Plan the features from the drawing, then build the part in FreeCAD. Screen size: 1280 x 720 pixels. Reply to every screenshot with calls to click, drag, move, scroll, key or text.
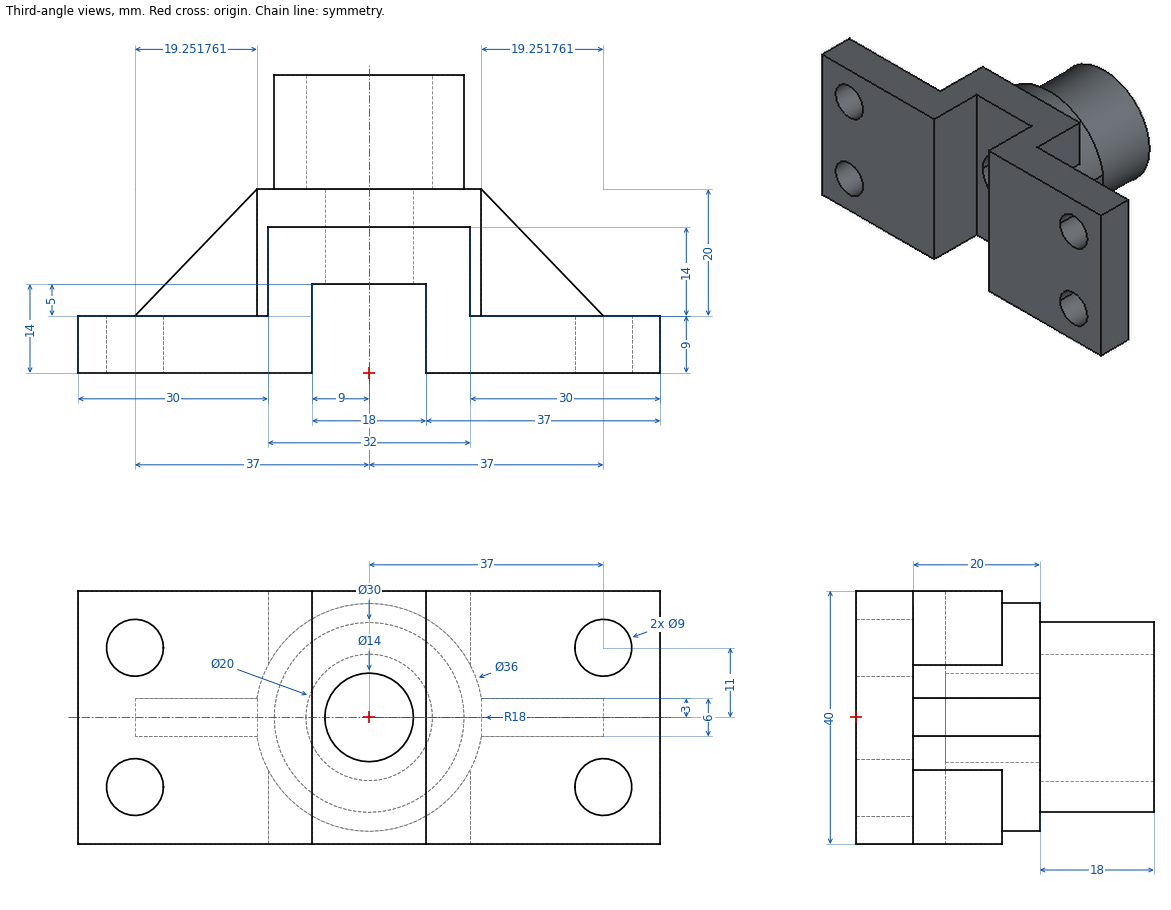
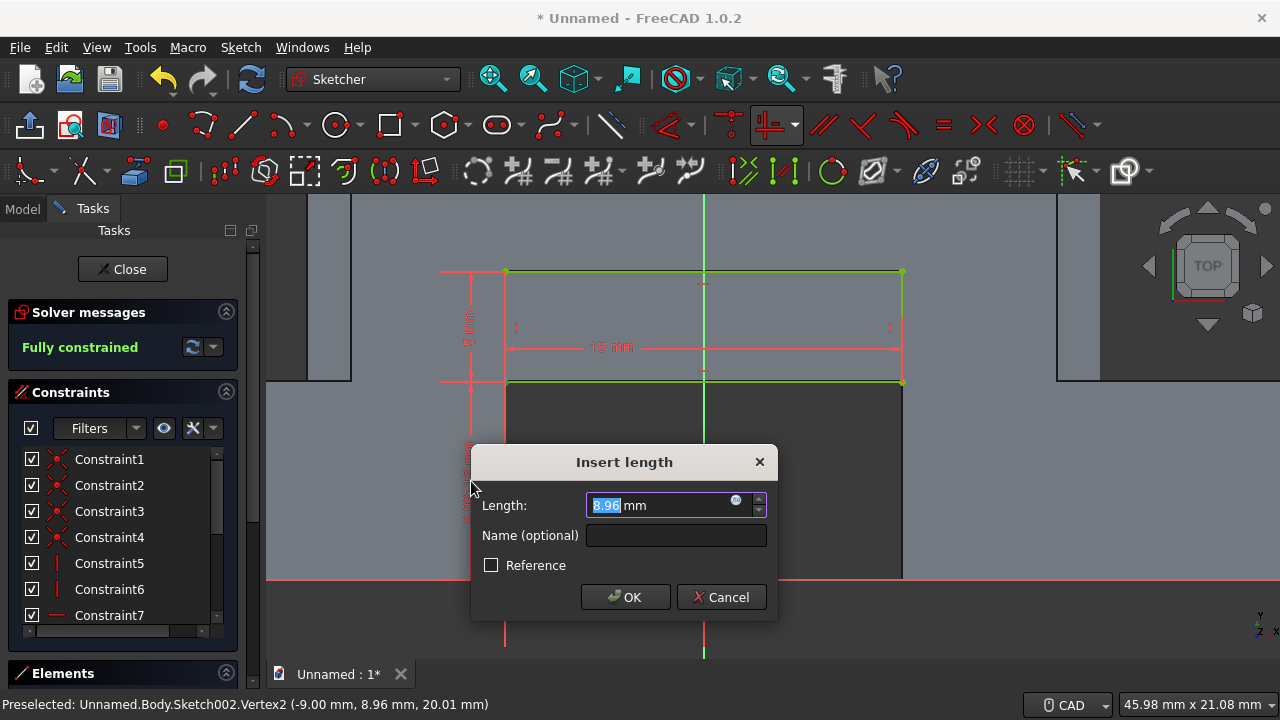
text(9)
key(Return)
key(Escape)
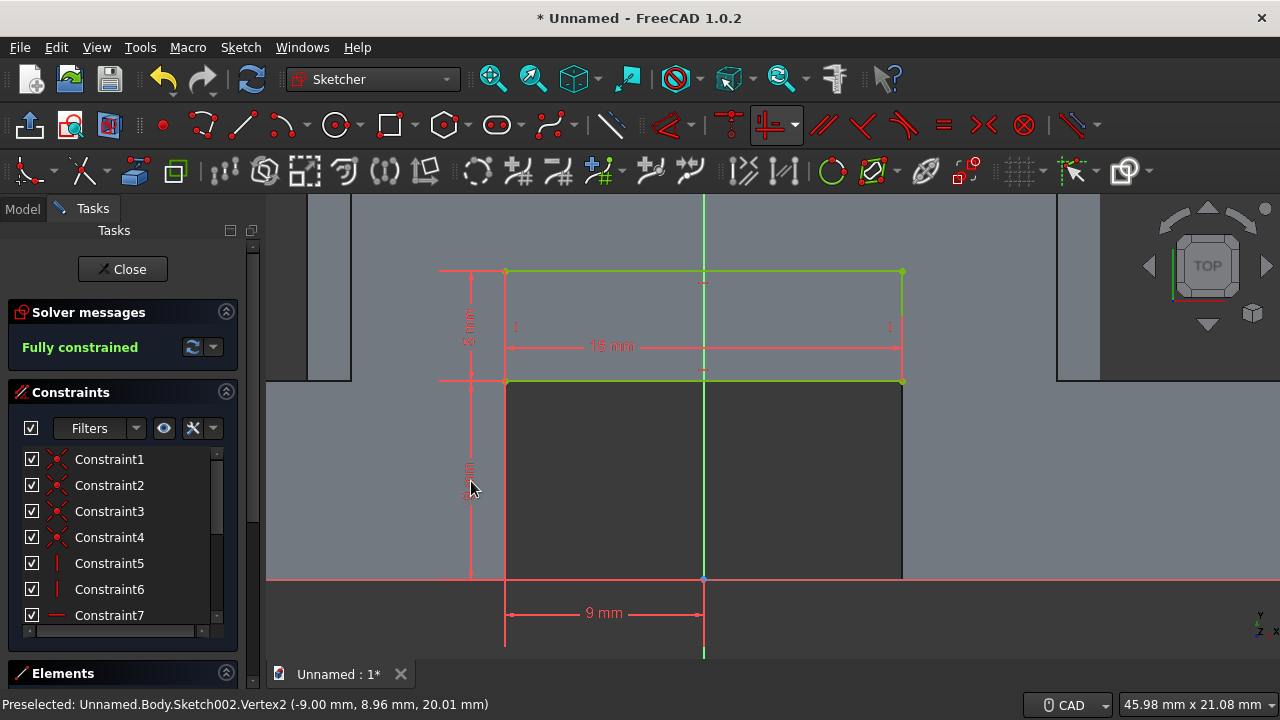
click(123, 269)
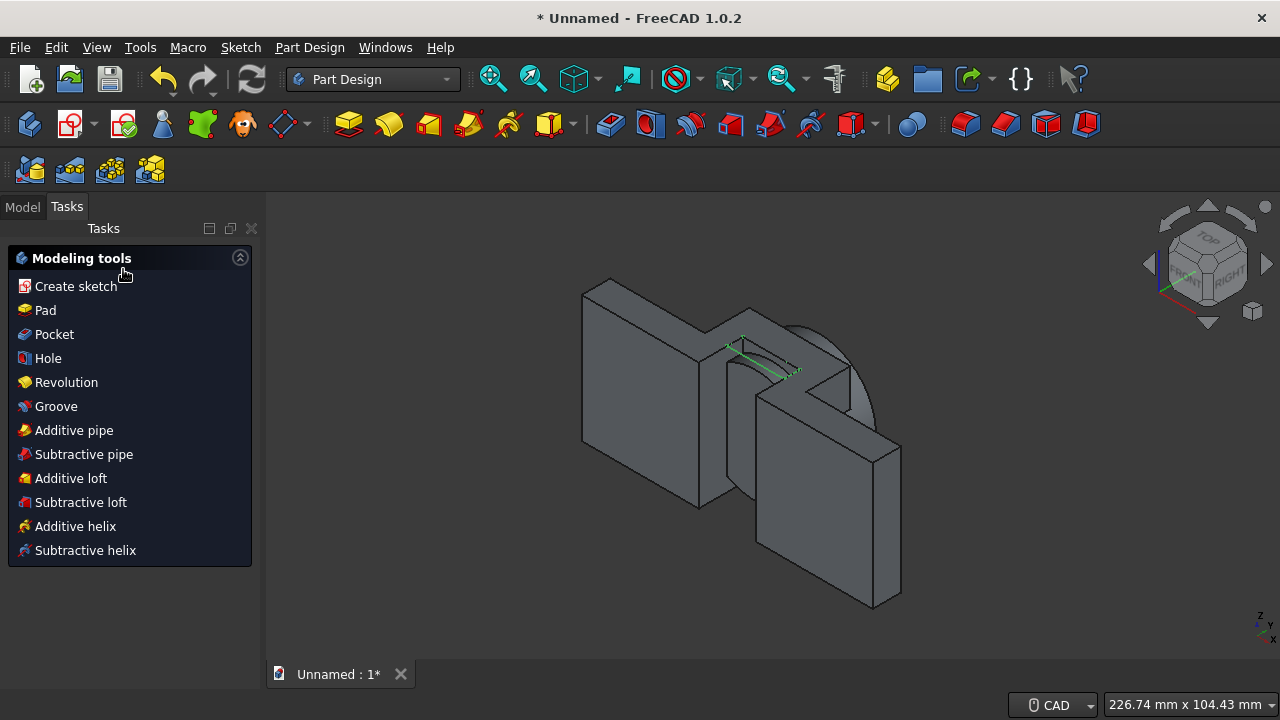
click(612, 124)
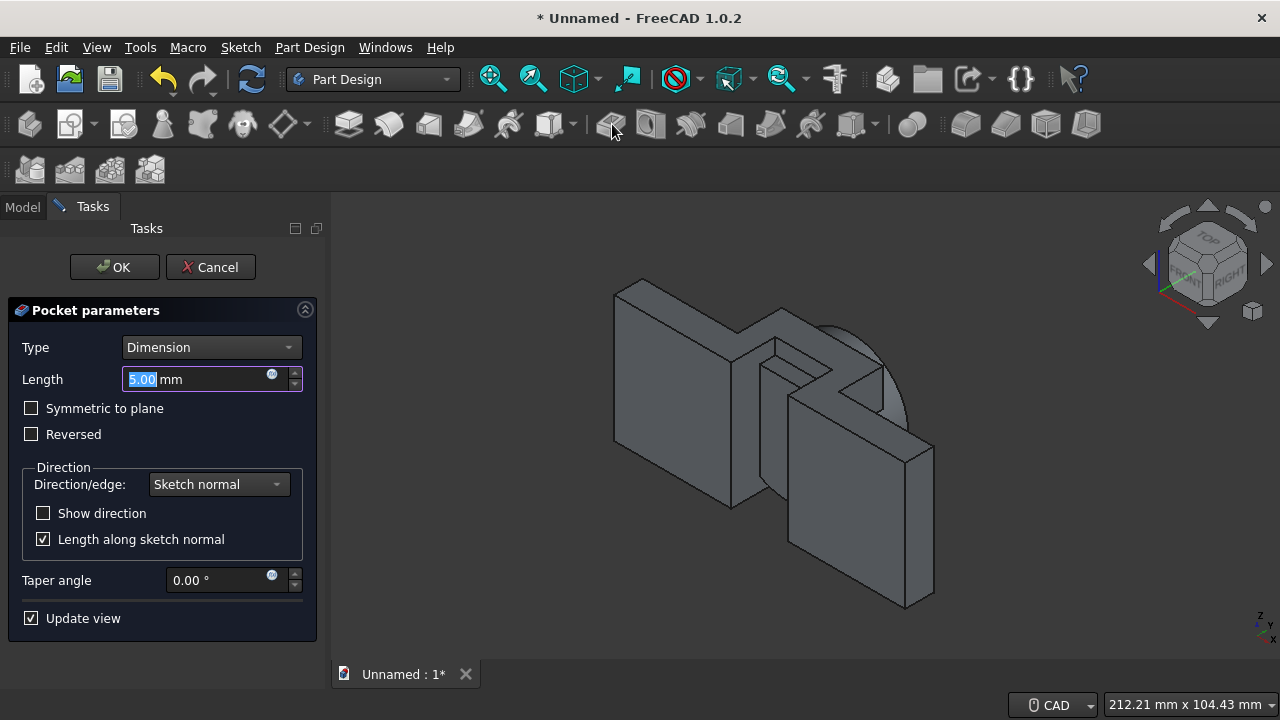
click(212, 348)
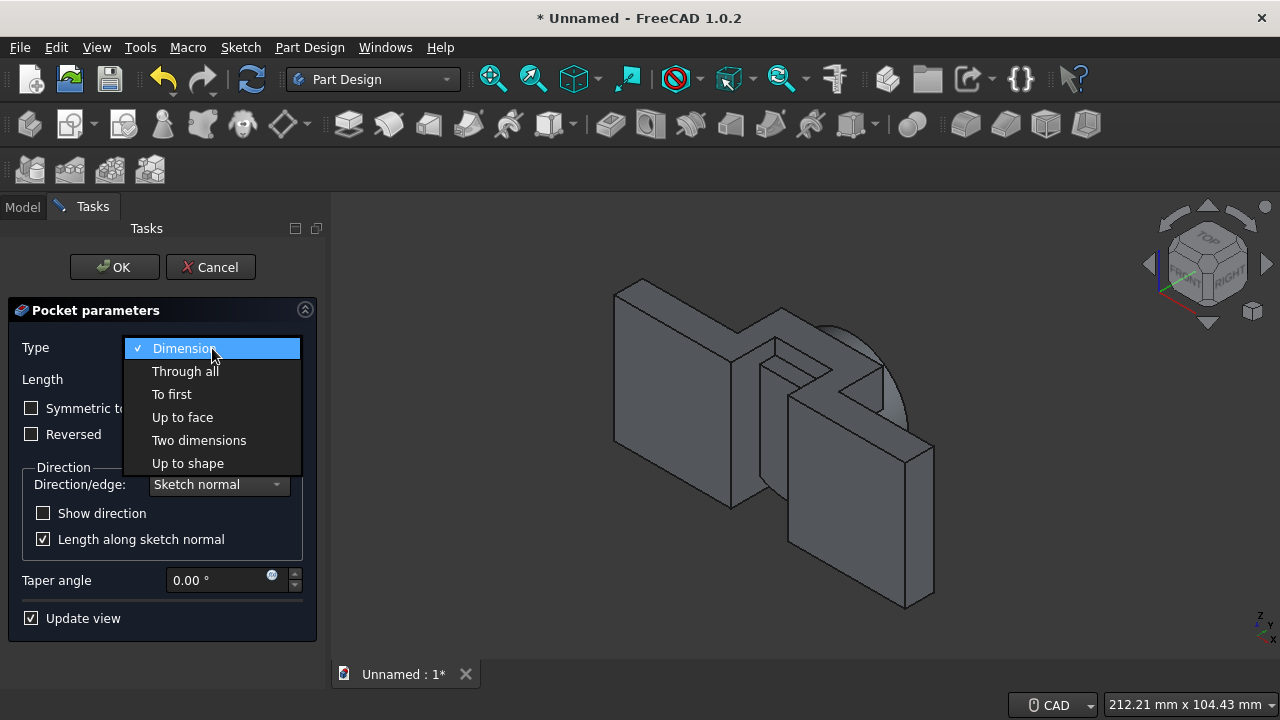
click(212, 372)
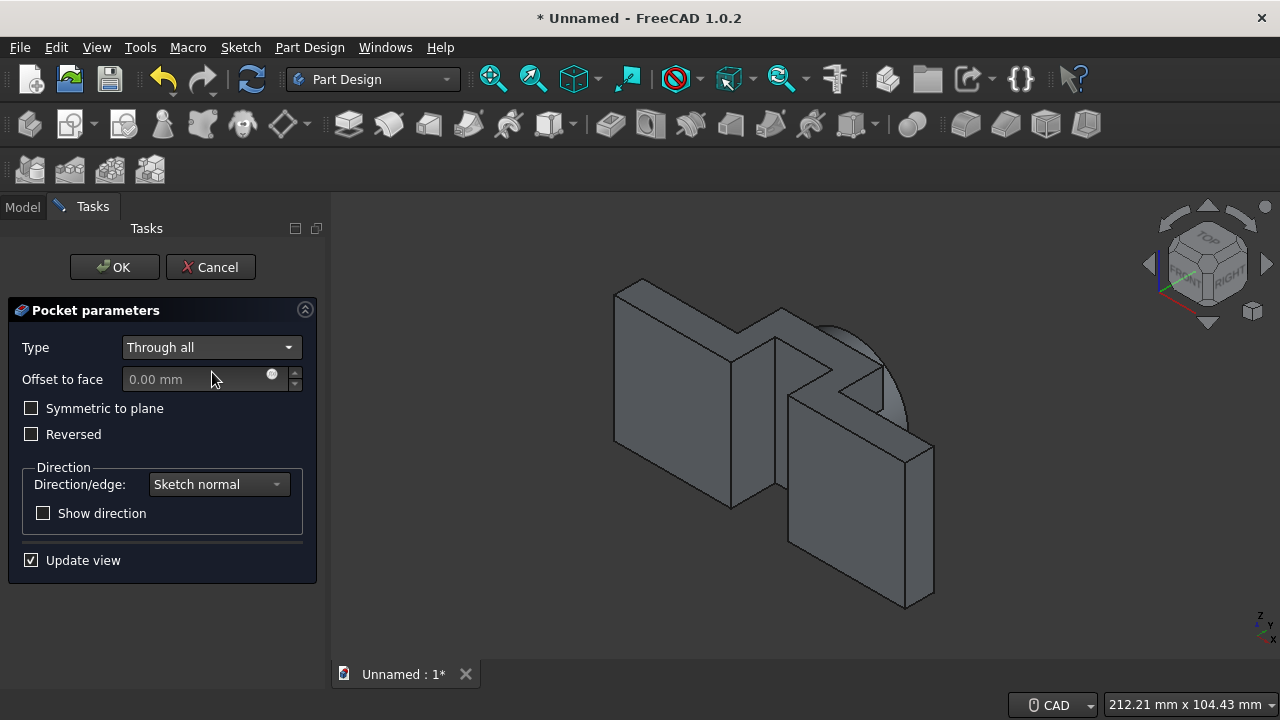
click(115, 267)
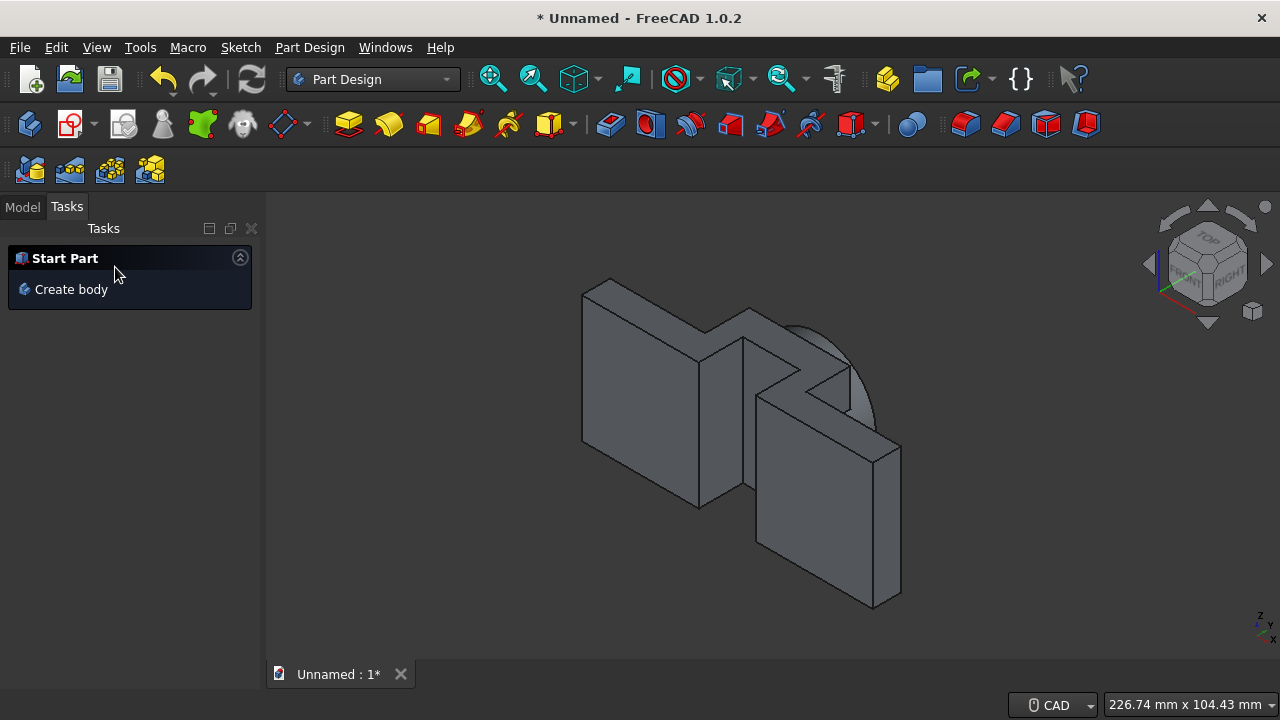
key(4)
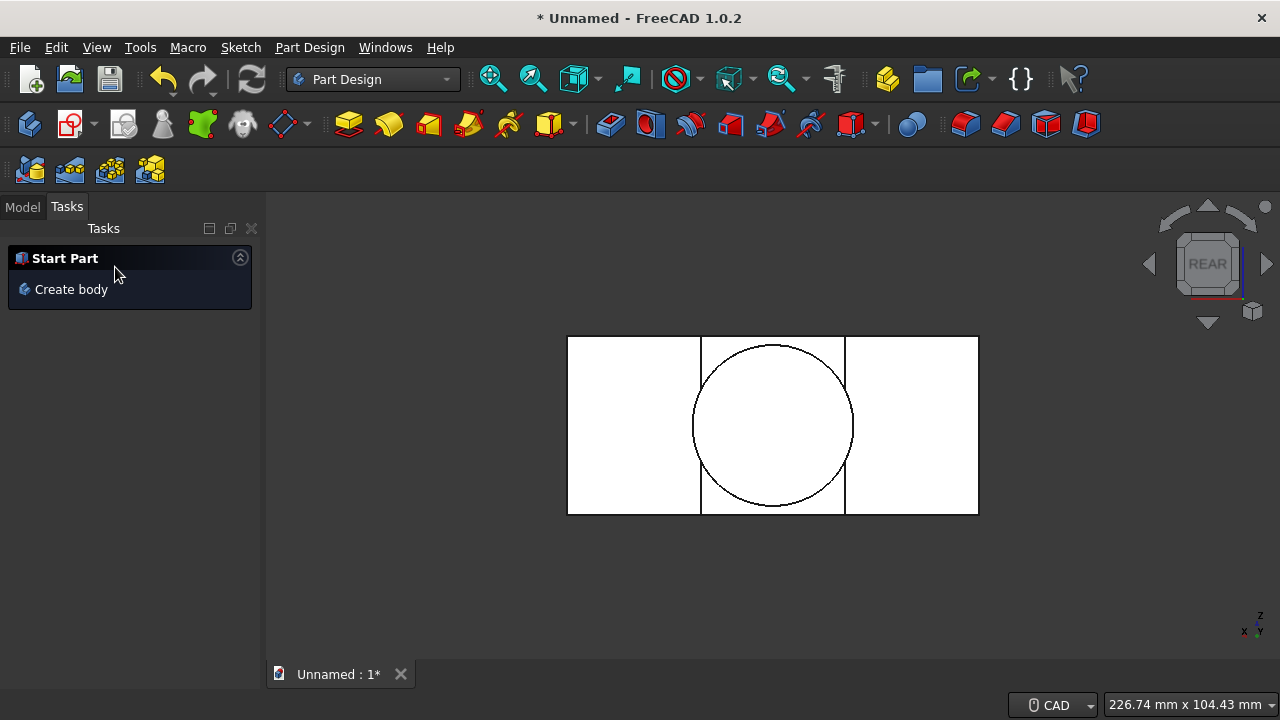
key(v)
key(f)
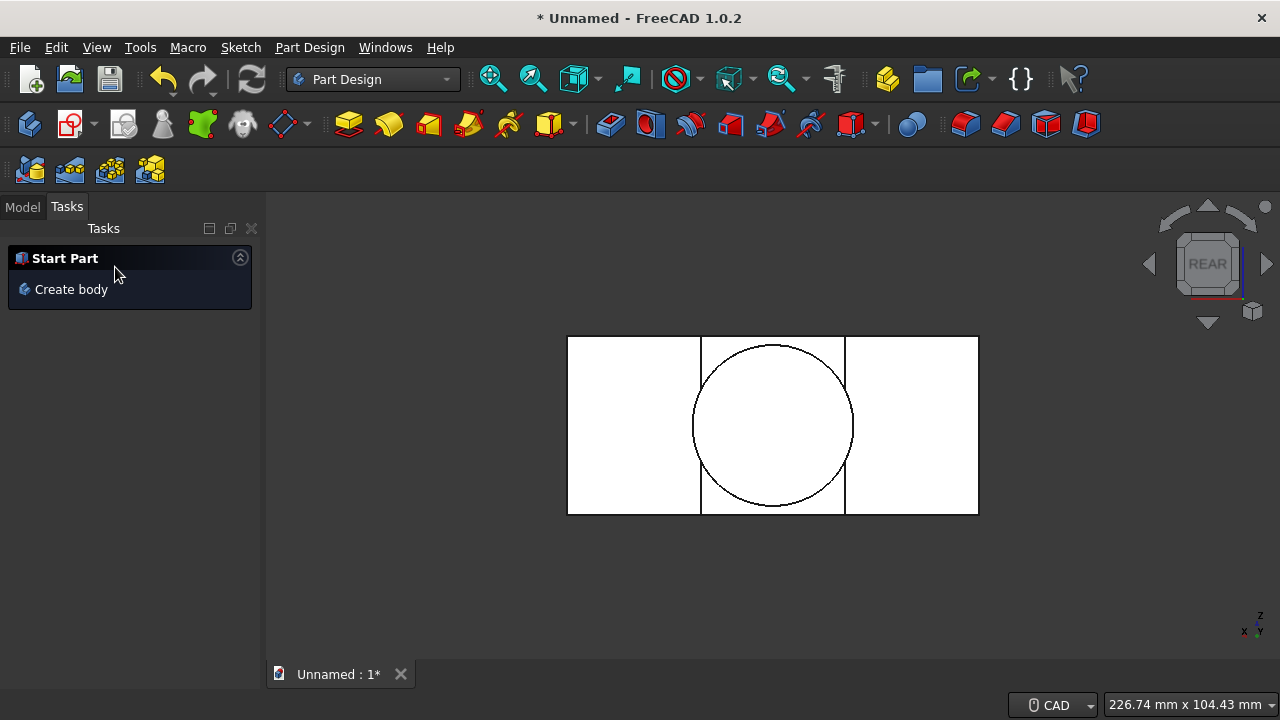
click(773, 425)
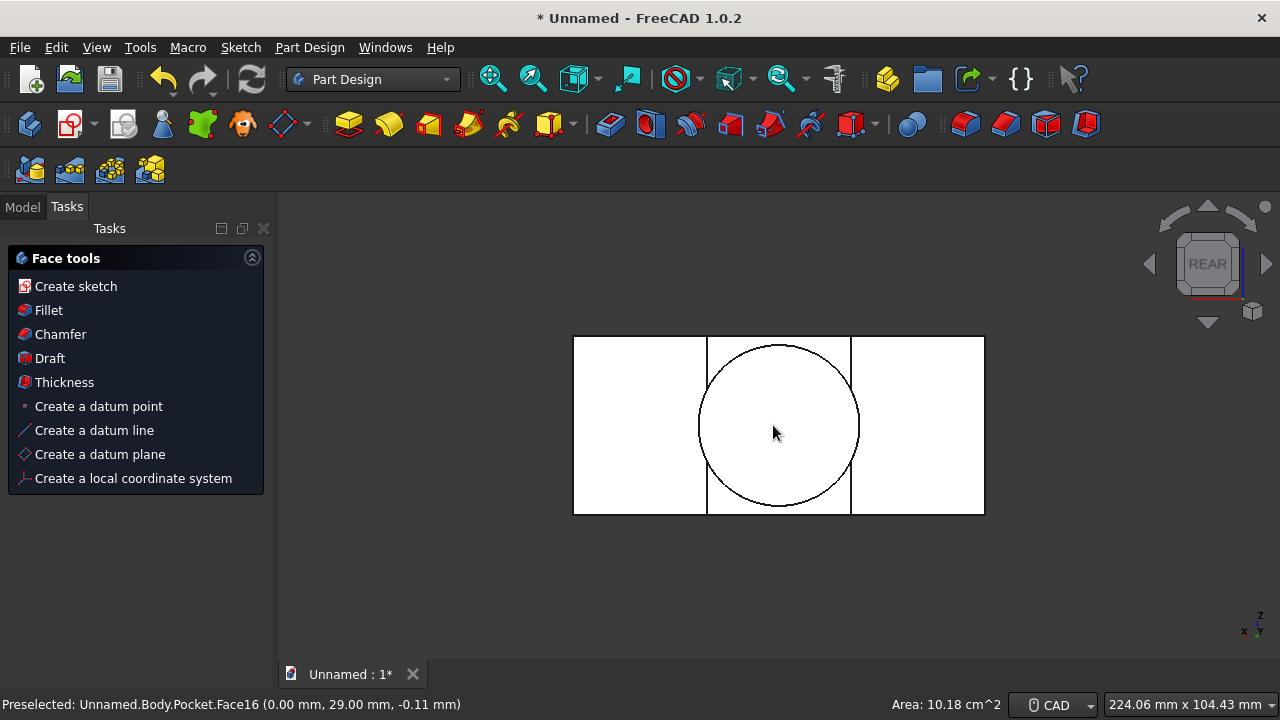
click(70, 124)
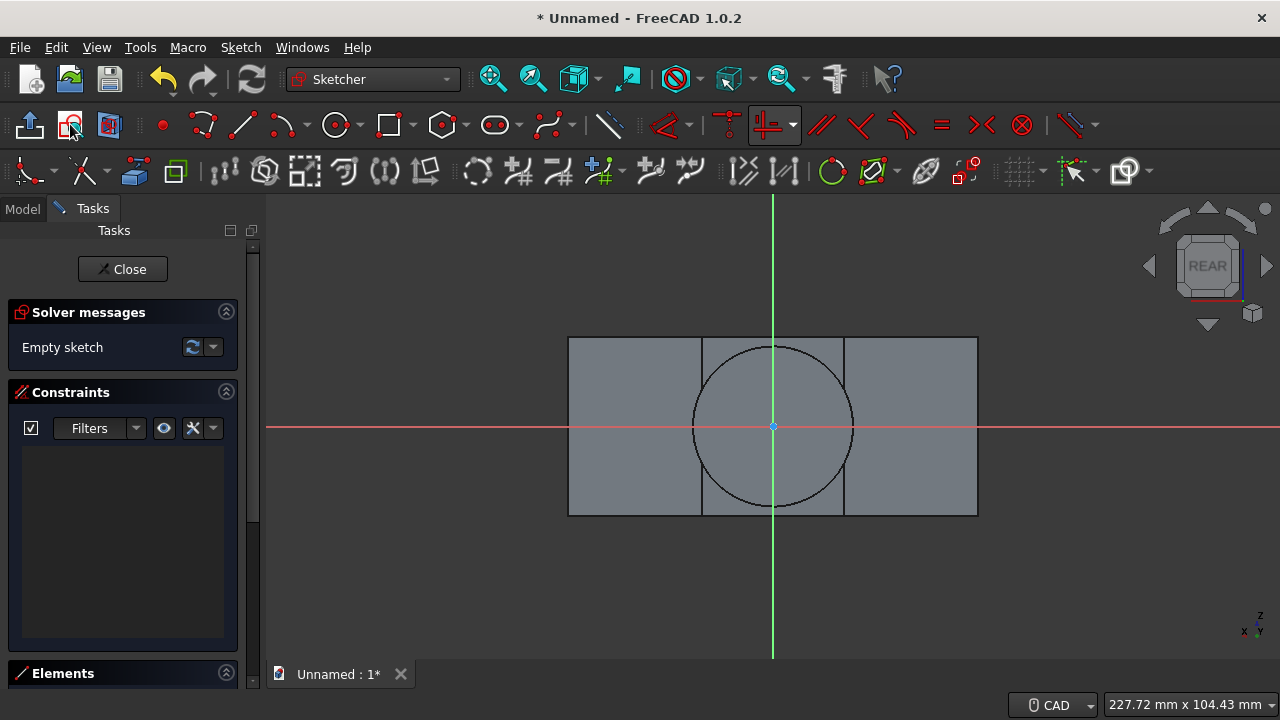
scroll(829, 427, up, 4)